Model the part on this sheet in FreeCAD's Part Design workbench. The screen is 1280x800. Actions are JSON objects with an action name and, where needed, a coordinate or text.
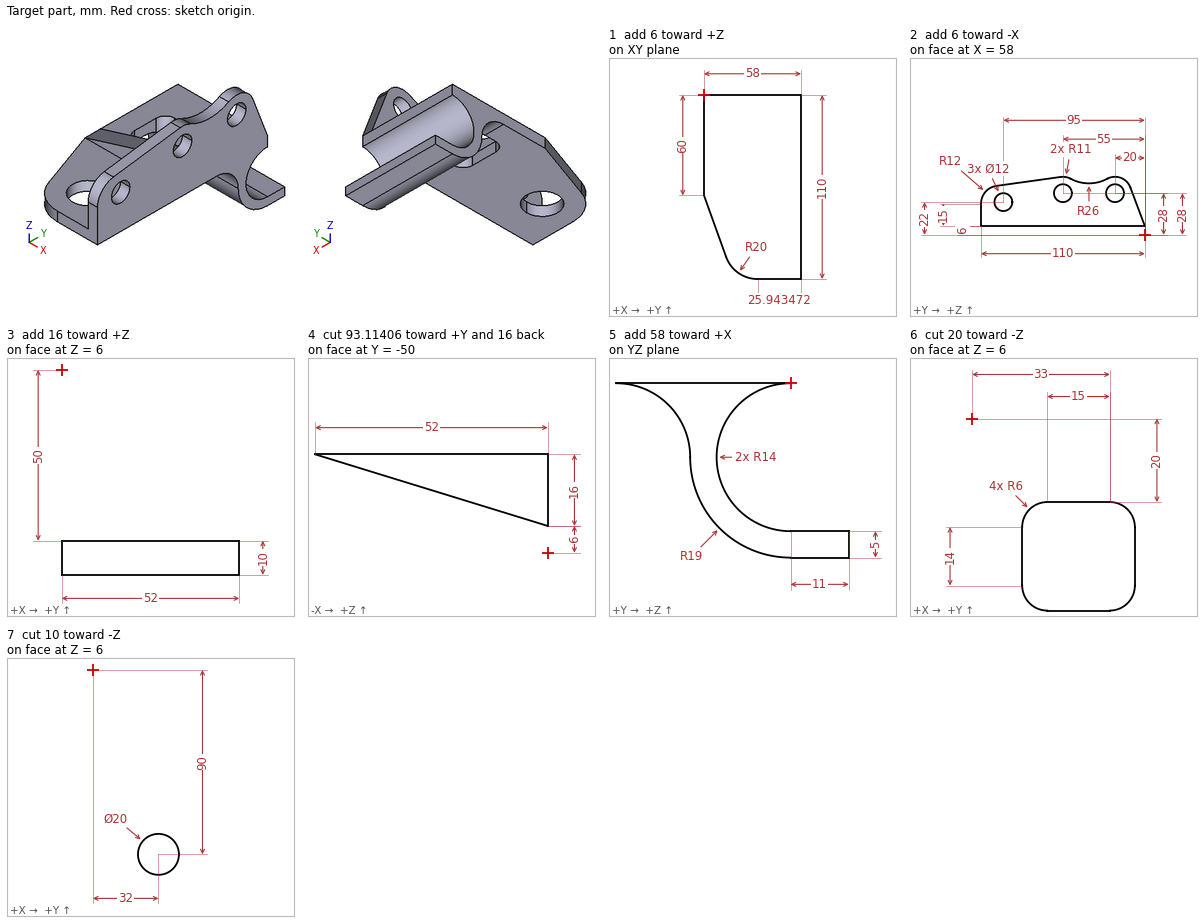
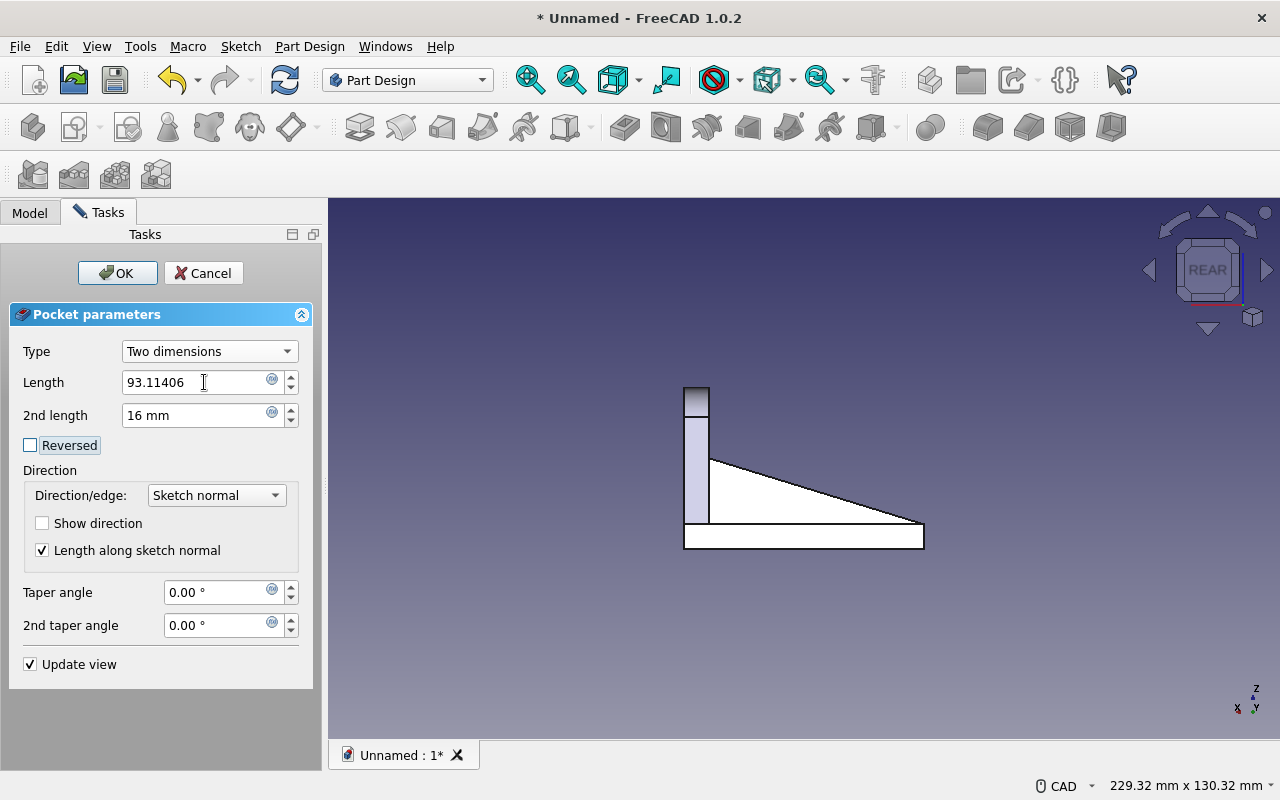
{"action": "left_click", "coordinate": [31, 445]}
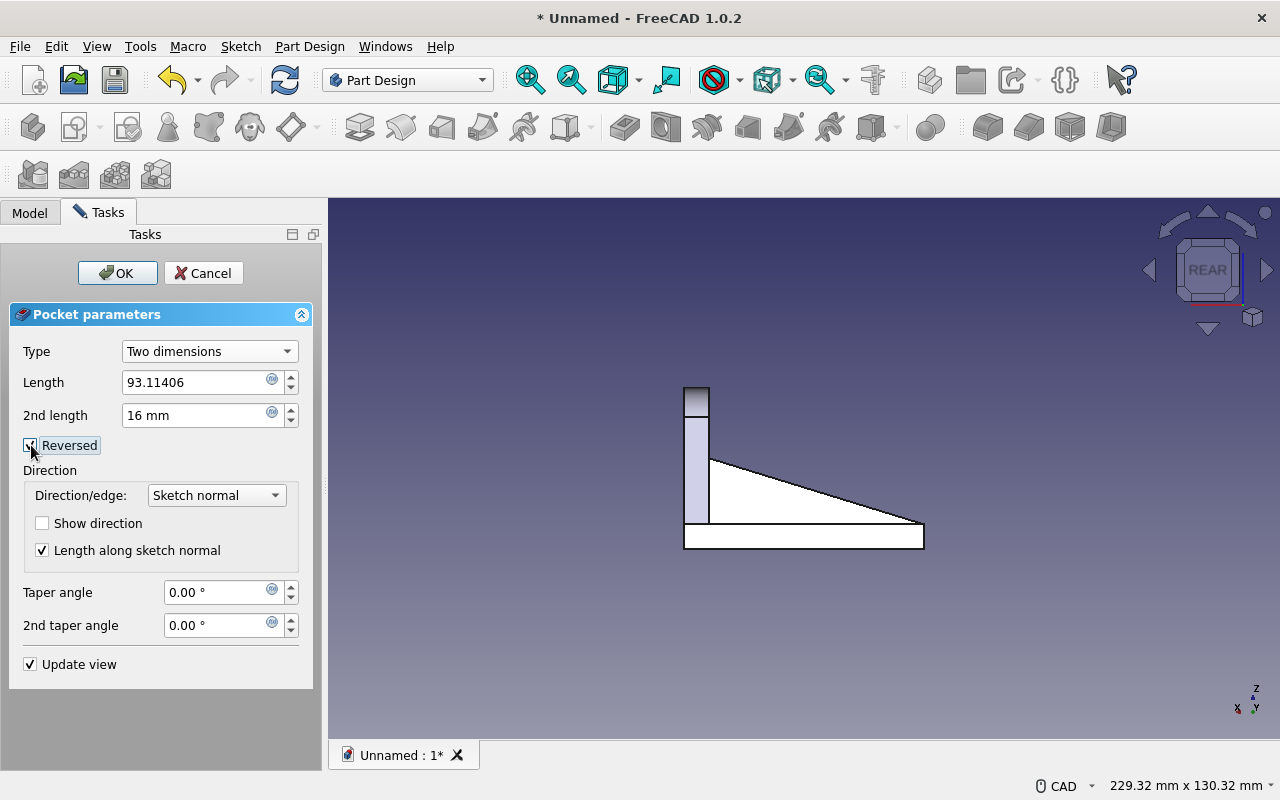
{"action": "left_click", "coordinate": [118, 273]}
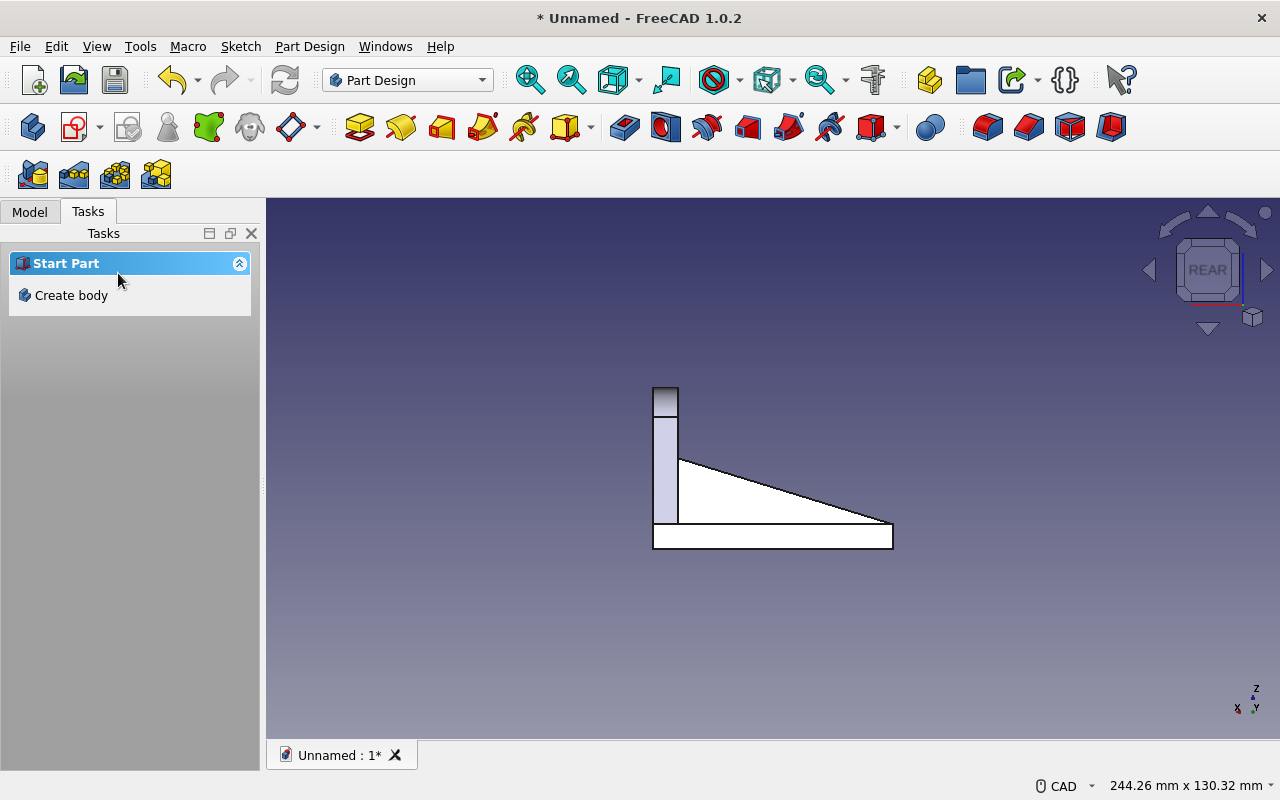
{"action": "key", "text": "v f"}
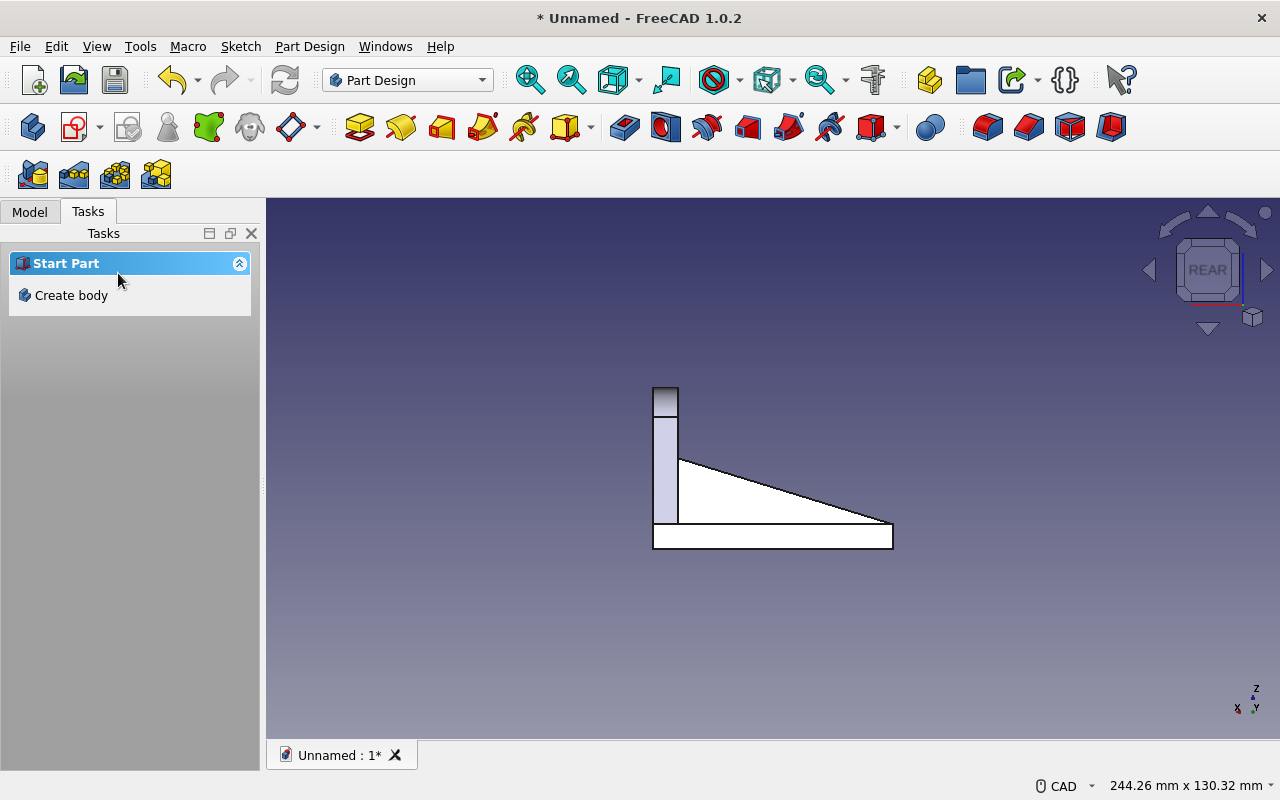
{"action": "left_click", "coordinate": [74, 128]}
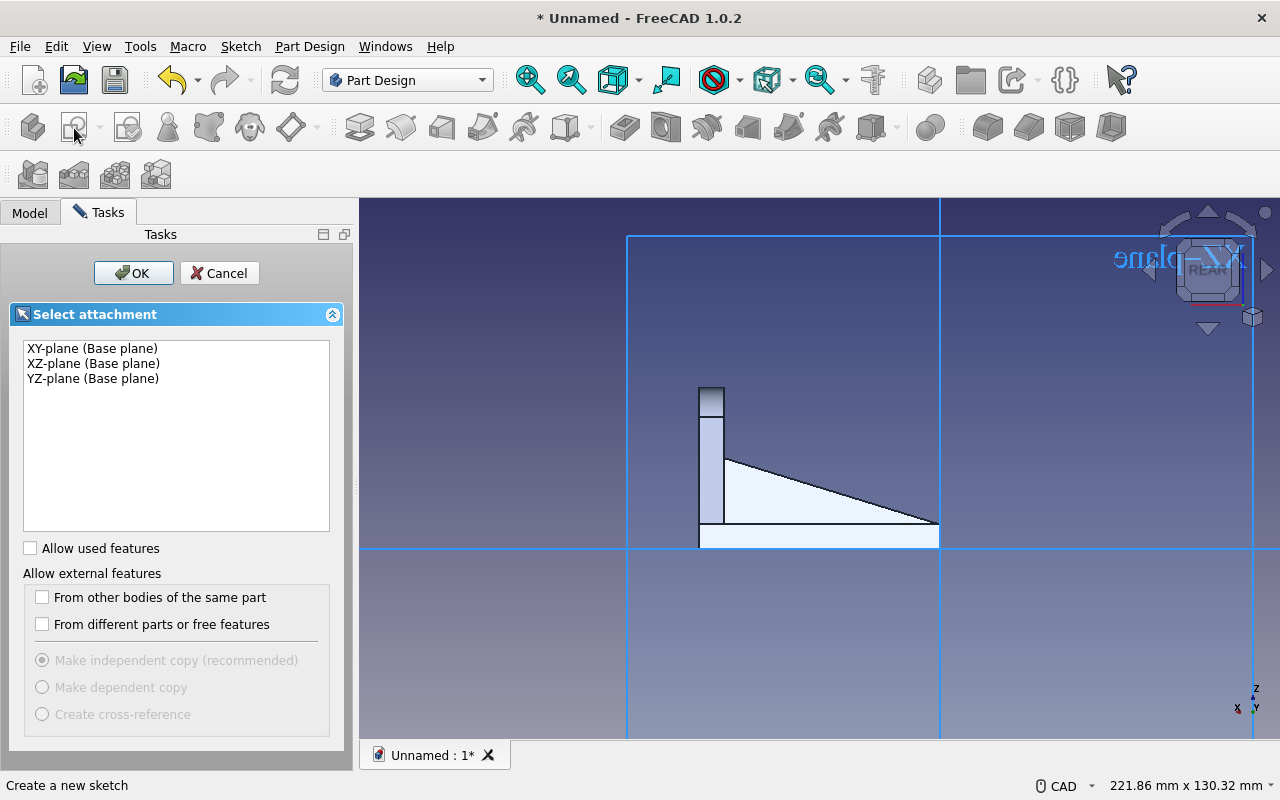
{"action": "left_click", "coordinate": [84, 378]}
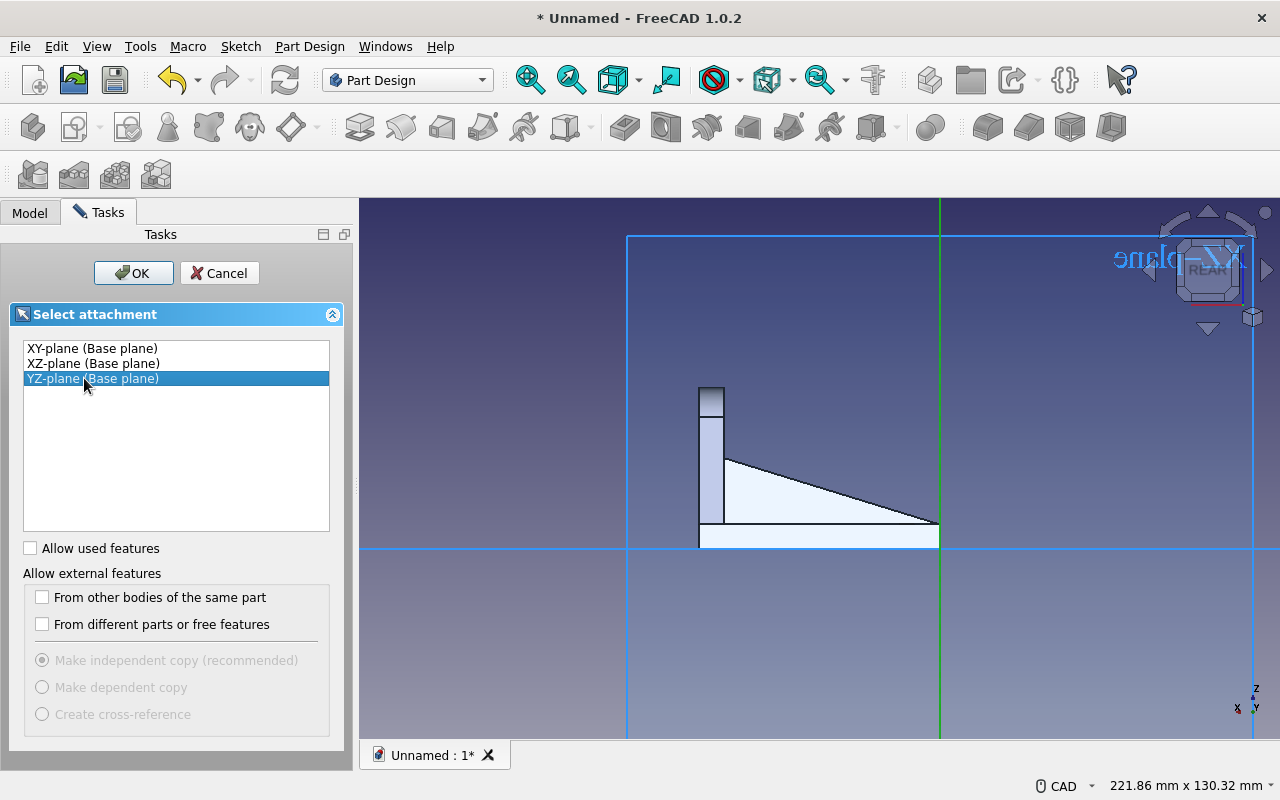
{"action": "left_click", "coordinate": [134, 273]}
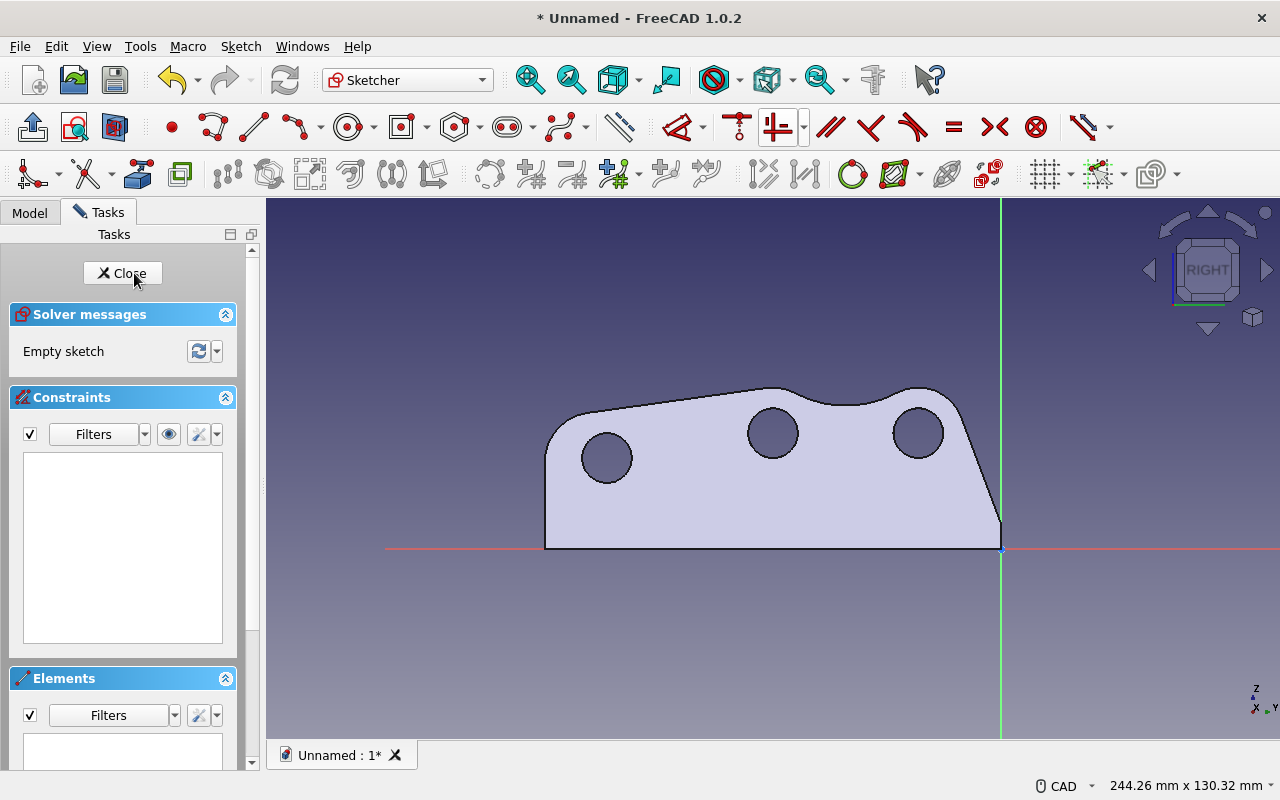
{"action": "left_click", "coordinate": [115, 128]}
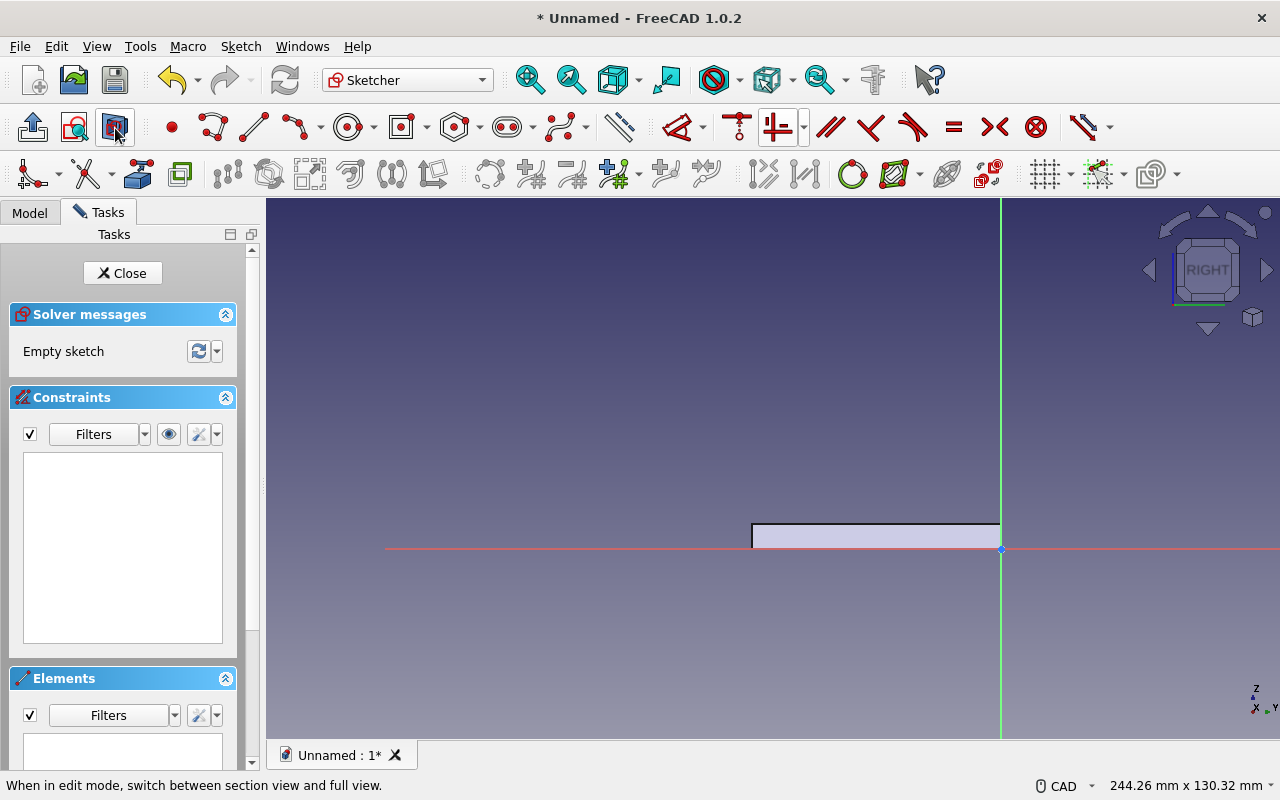
{"action": "scroll", "coordinate": [1102, 705], "scroll_direction": "up", "scroll_amount": 5}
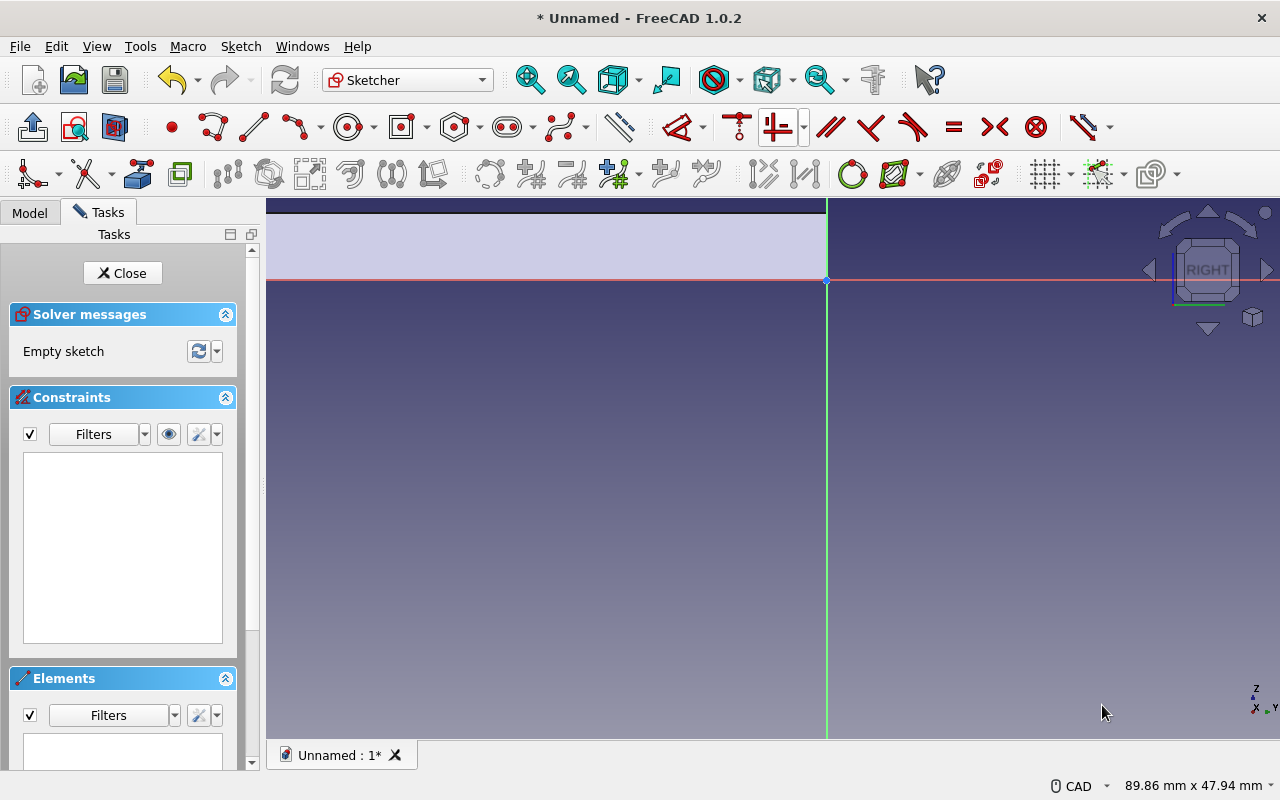
{"action": "left_click", "coordinate": [254, 128]}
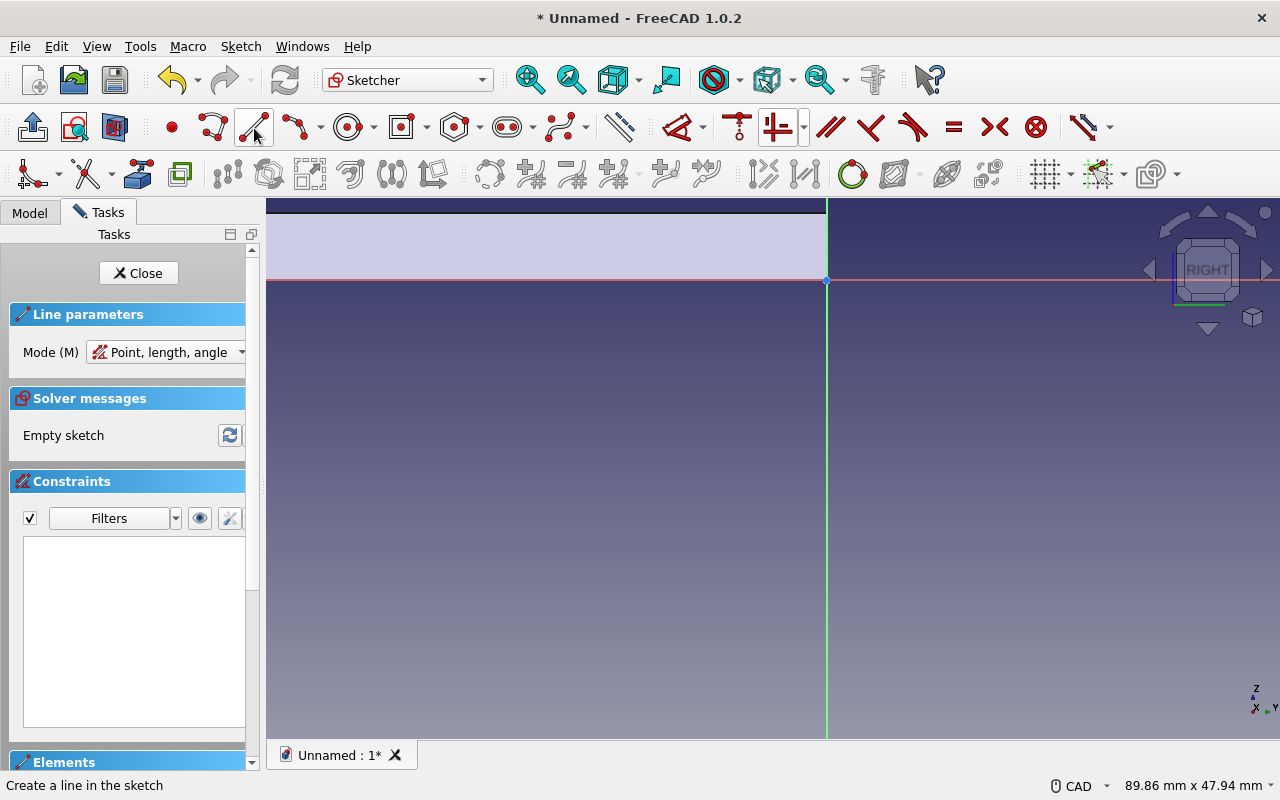
{"action": "left_click", "coordinate": [455, 280]}
{"action": "left_click", "coordinate": [827, 280]}